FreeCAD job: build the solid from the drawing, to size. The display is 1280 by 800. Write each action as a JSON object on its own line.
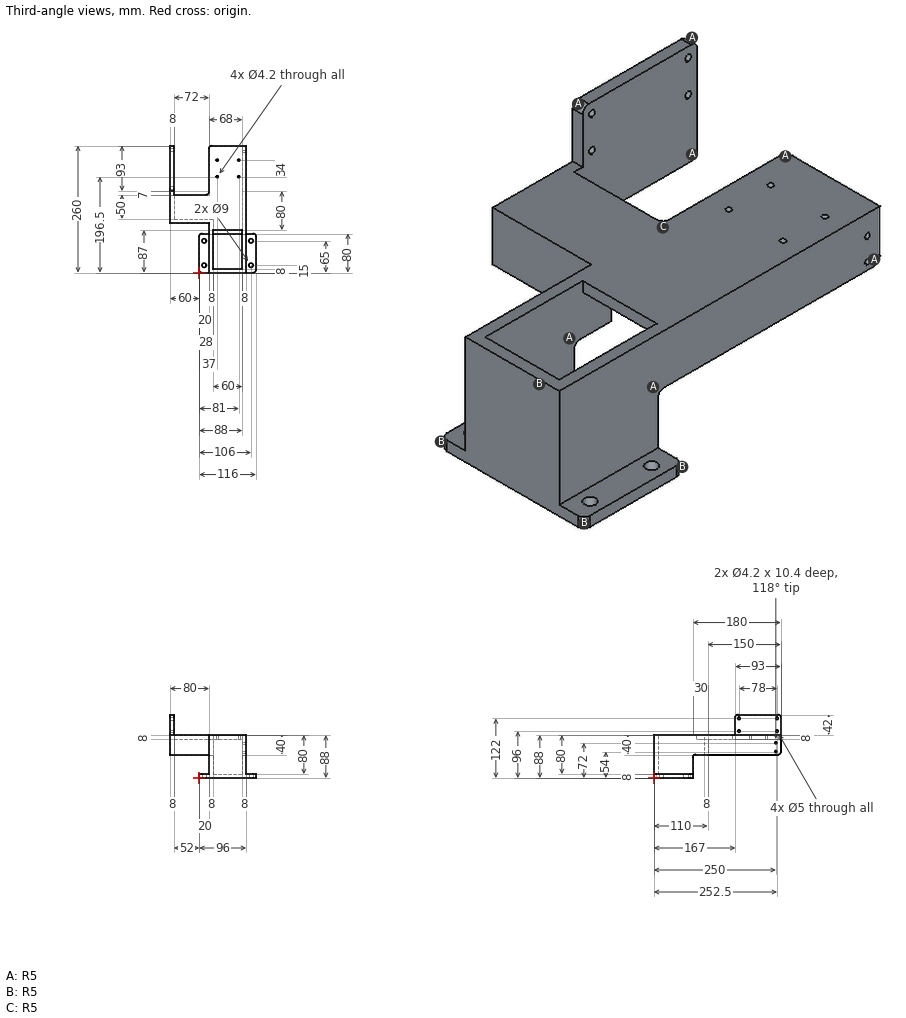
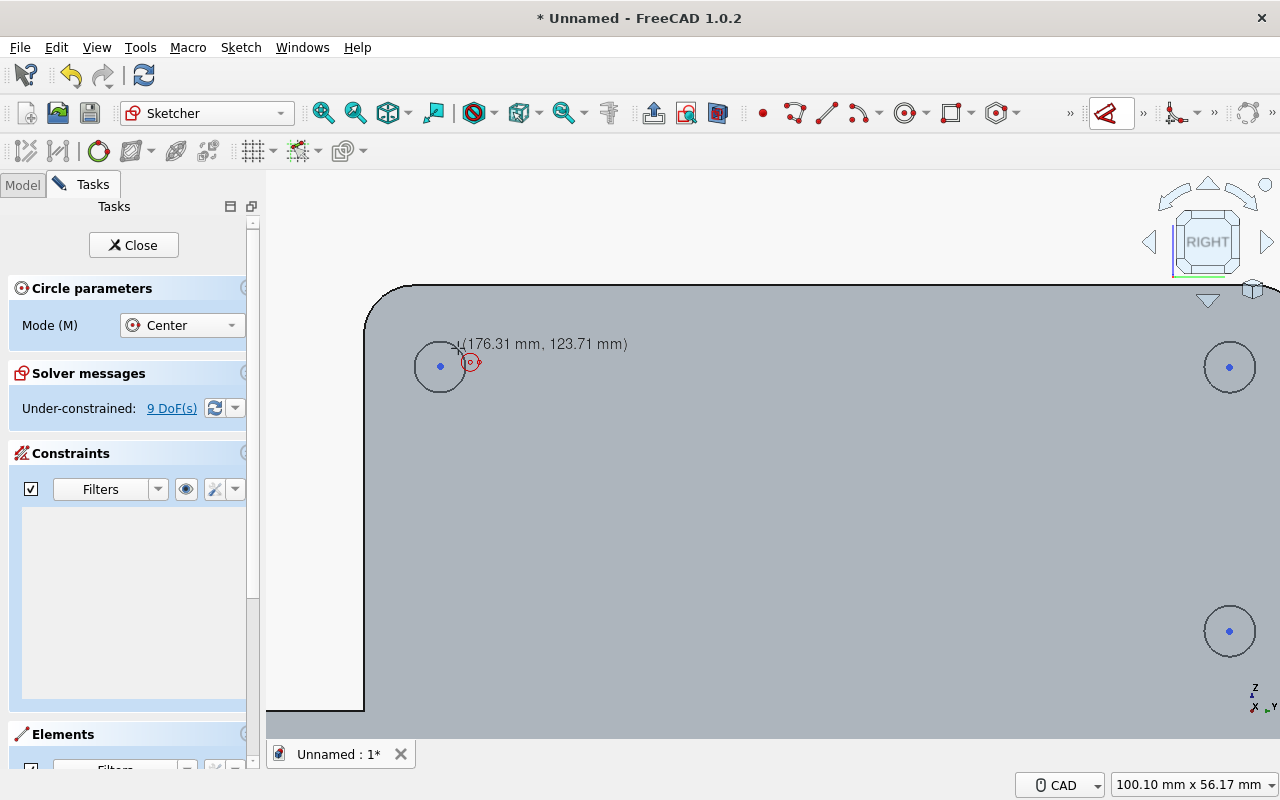
{"action": "left_click", "coordinate": [440, 630]}
{"action": "left_click", "coordinate": [458, 612]}
{"action": "key", "text": "Escape"}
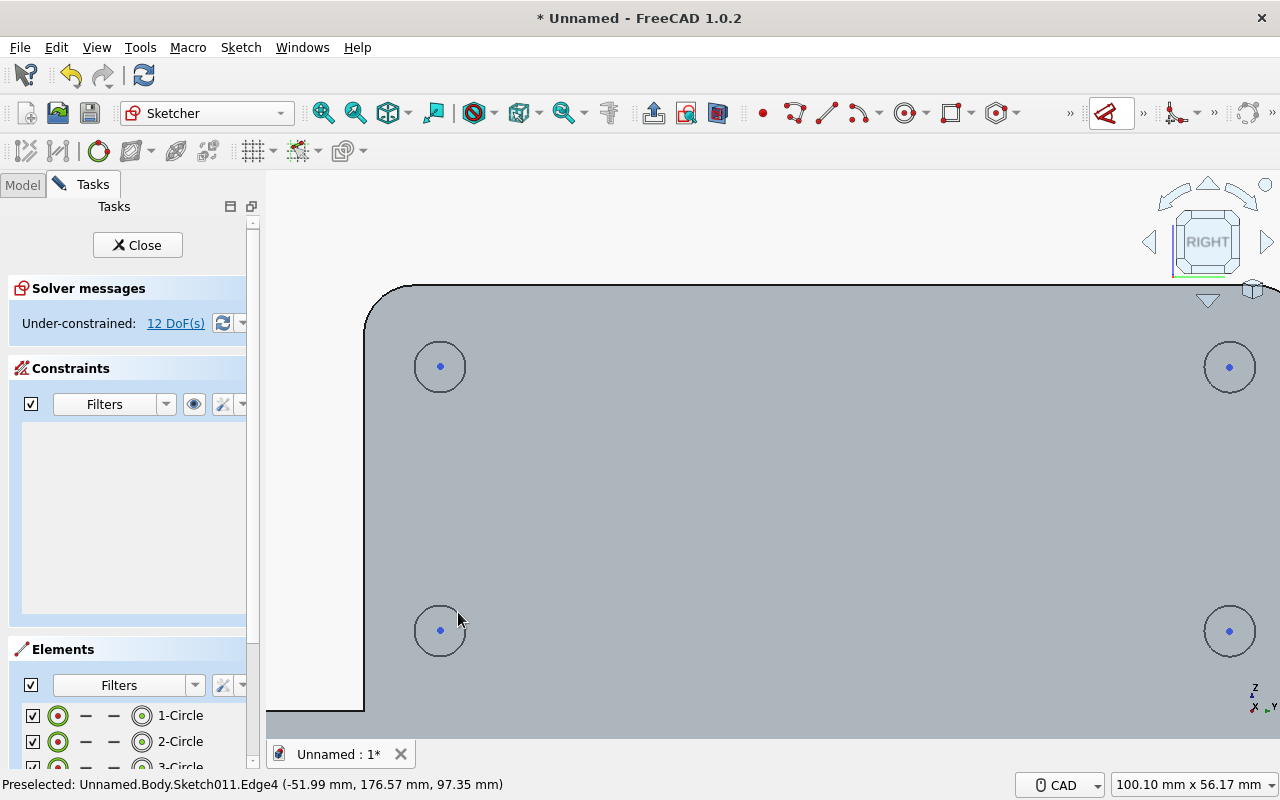
{"action": "scroll", "coordinate": [440, 366], "scroll_direction": "down", "scroll_amount": 2}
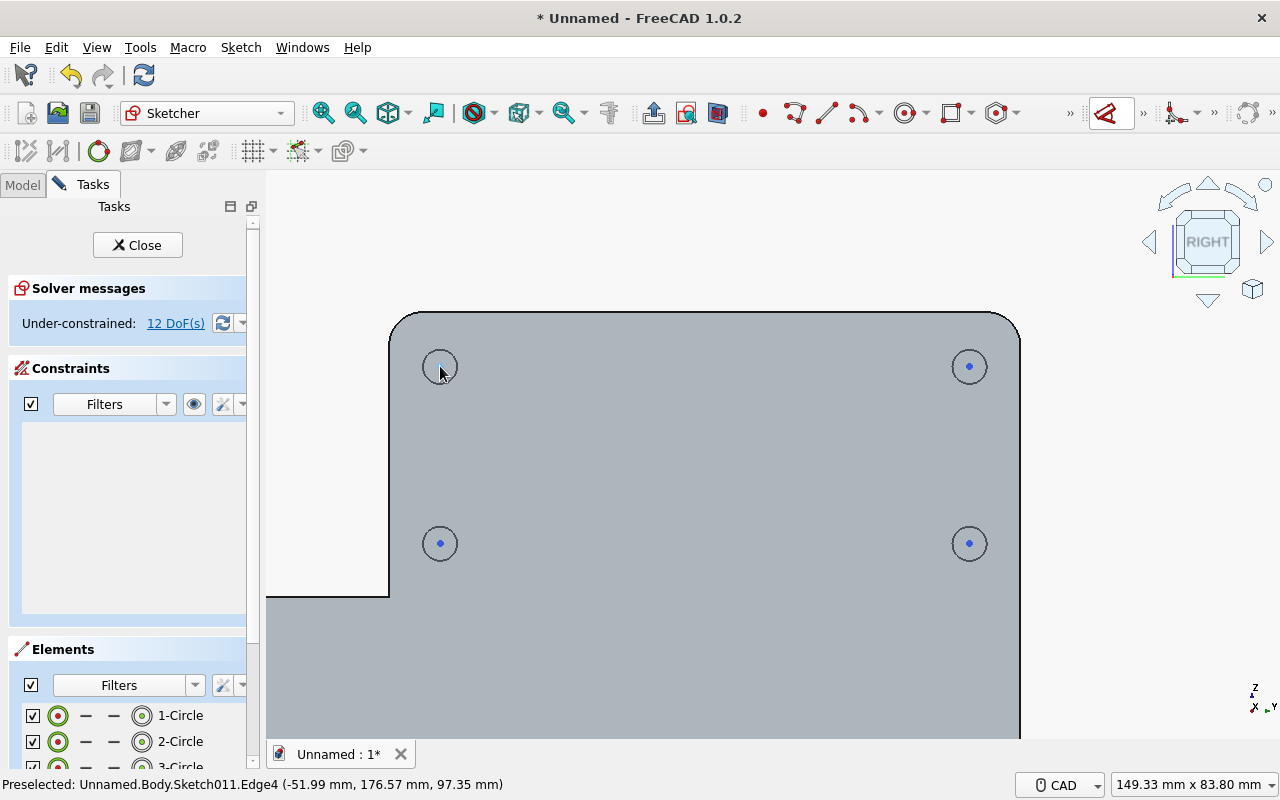
{"action": "left_click", "coordinate": [982, 532]}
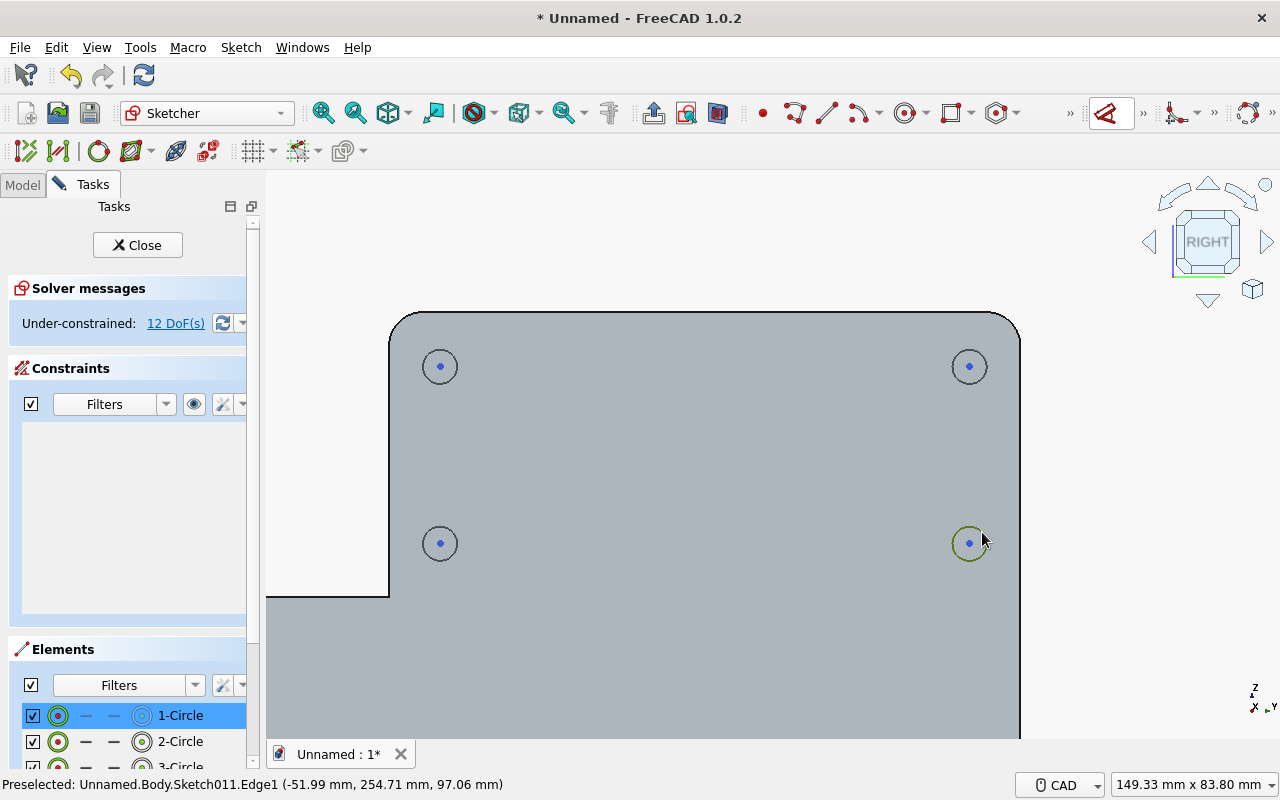
{"action": "left_click", "coordinate": [982, 355]}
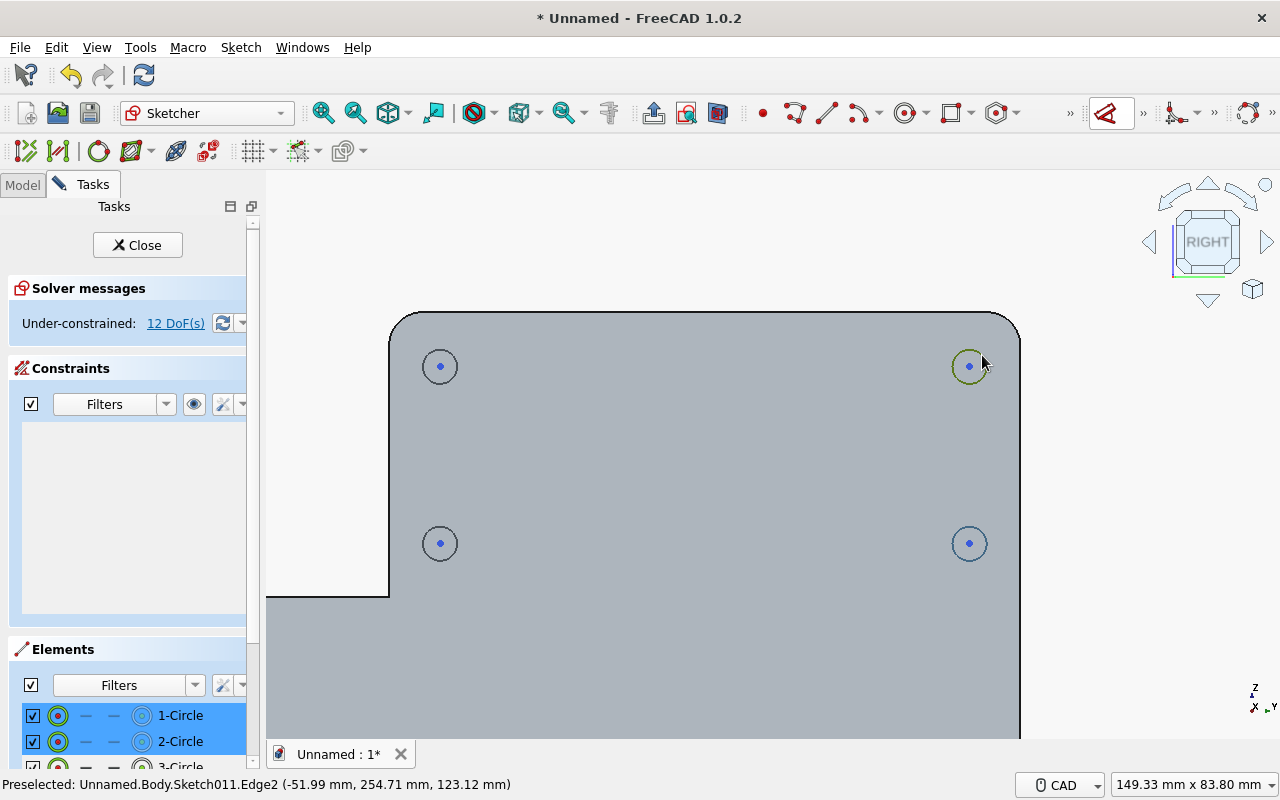
{"action": "left_click", "coordinate": [452, 355]}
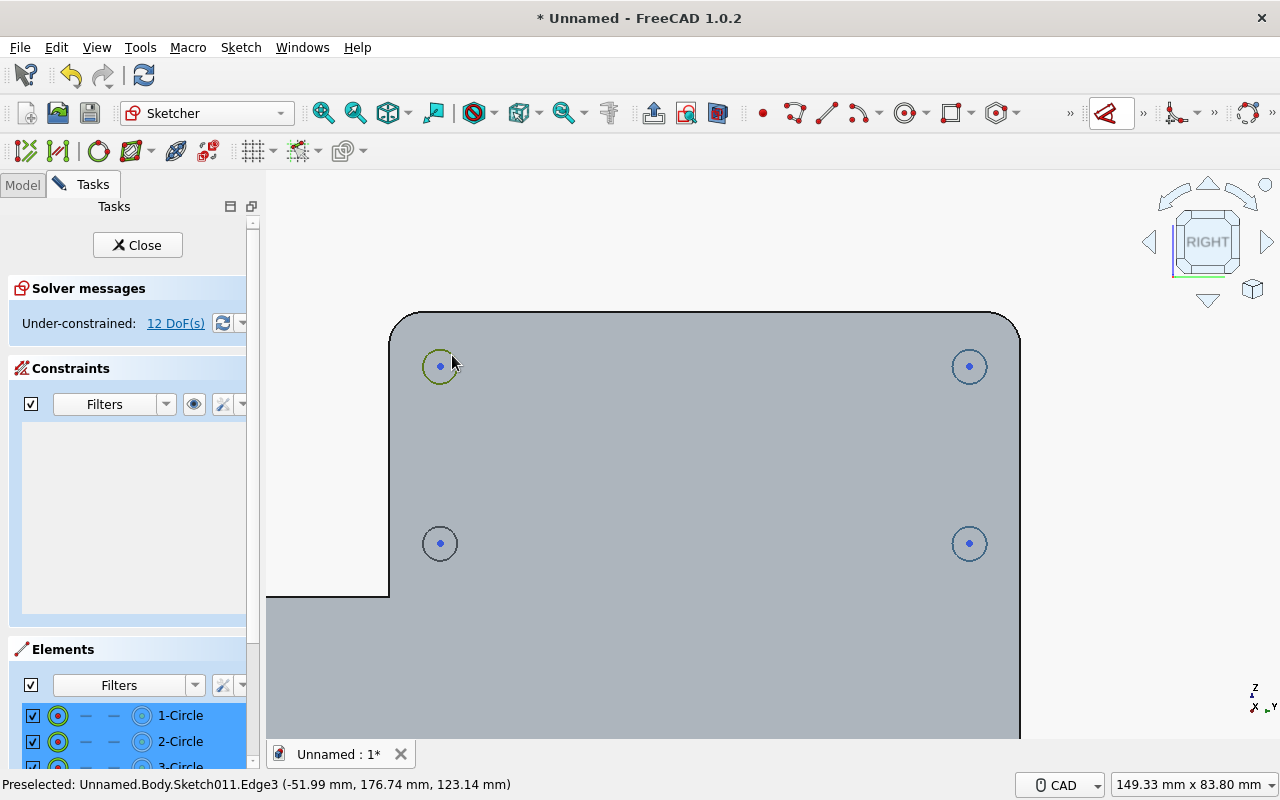
{"action": "left_click", "coordinate": [452, 532]}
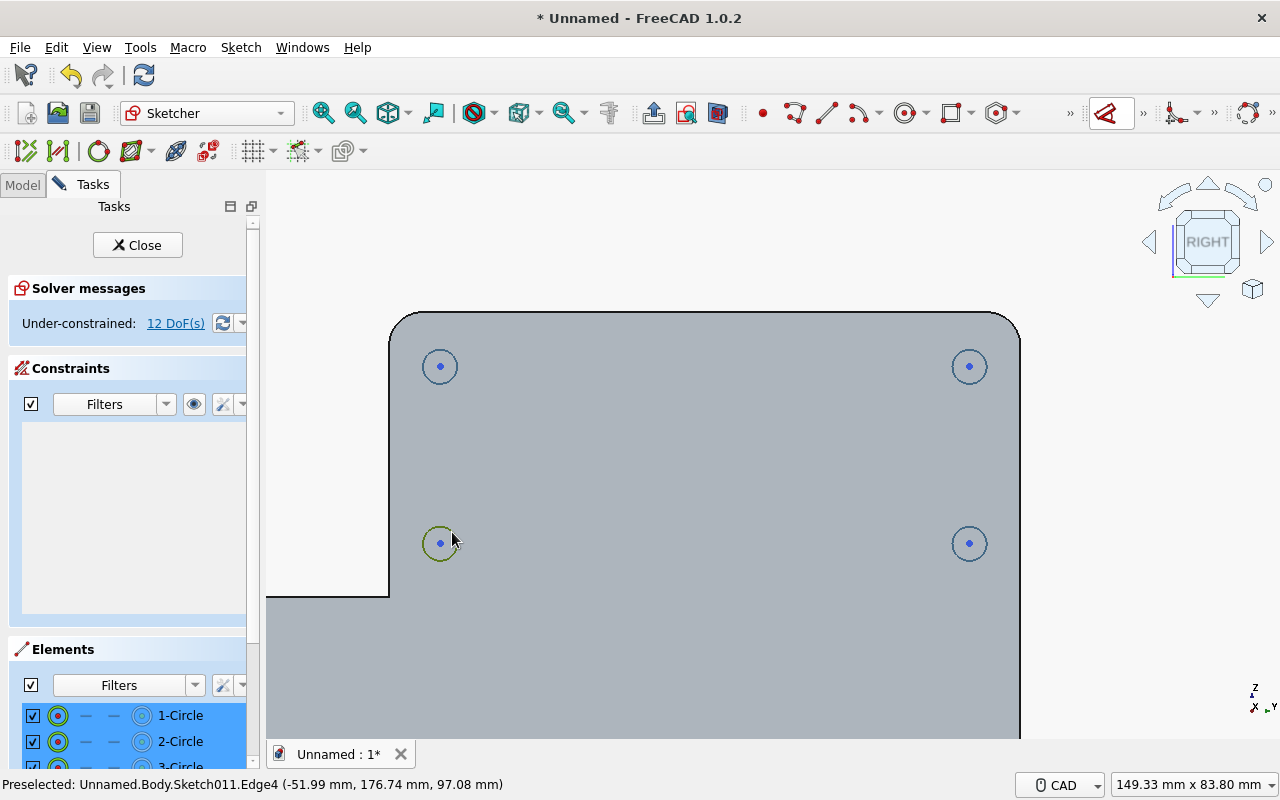
{"action": "key", "text": "e"}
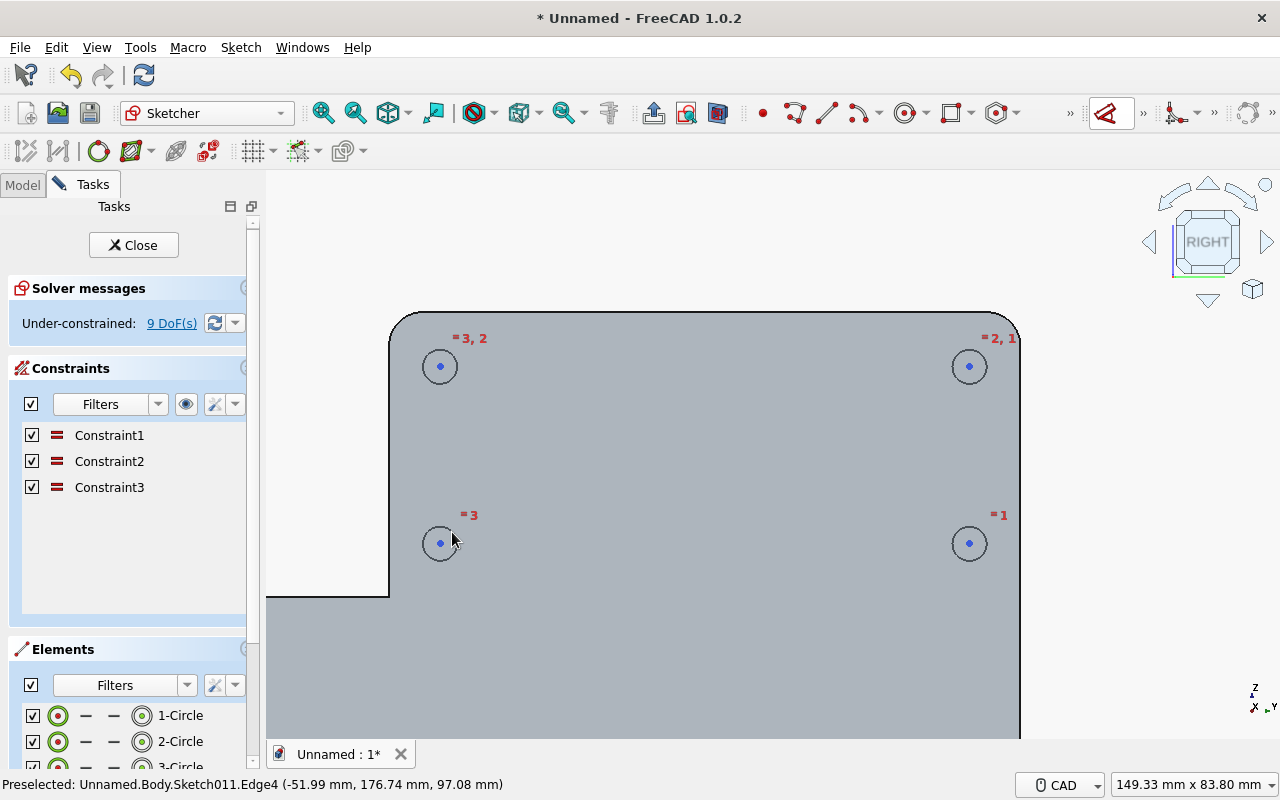
{"action": "left_click", "coordinate": [970, 544]}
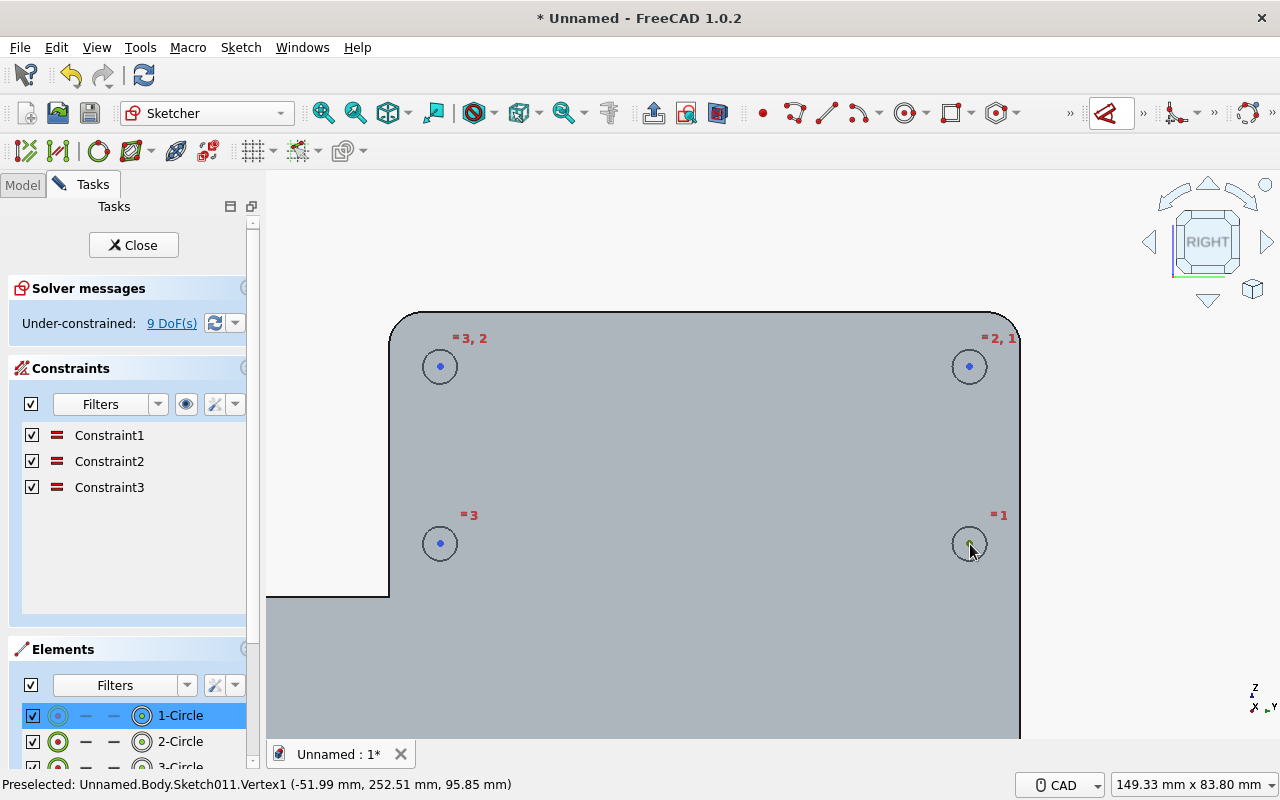
{"action": "left_click", "coordinate": [970, 367]}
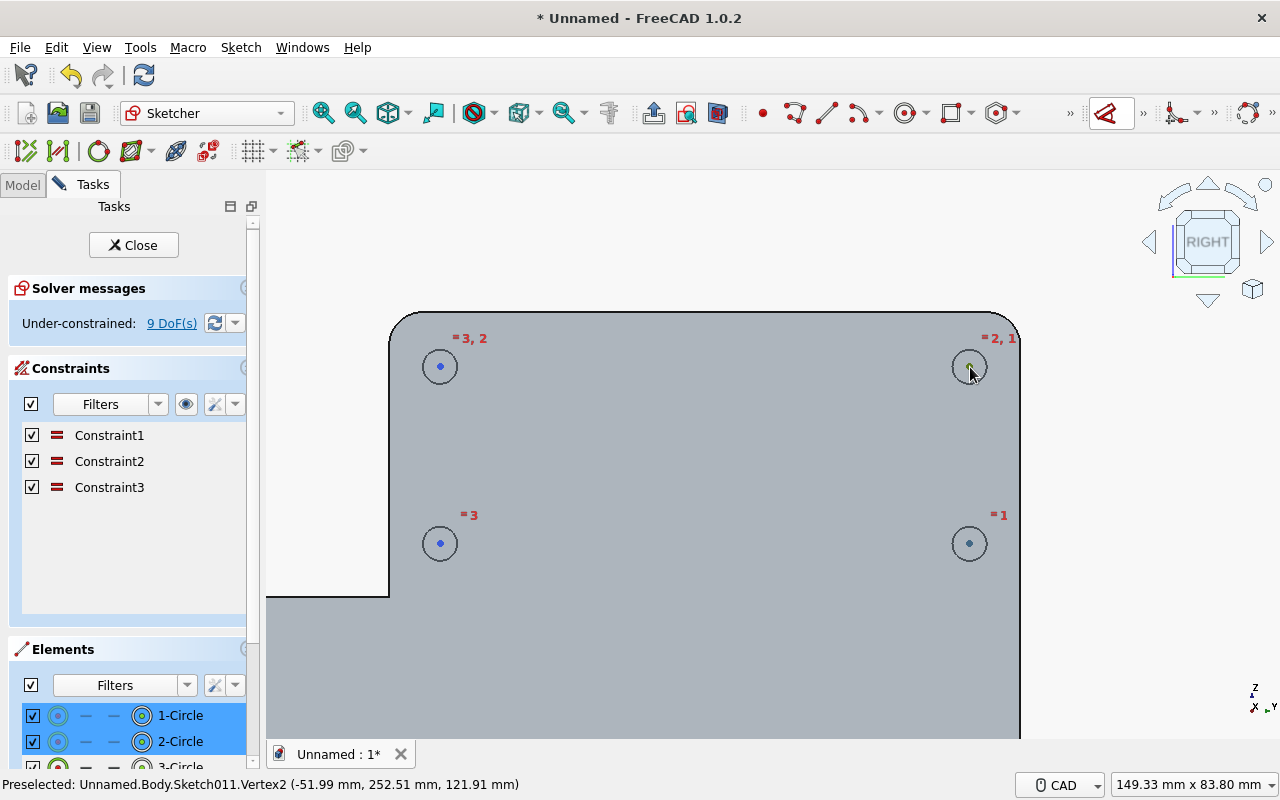
{"action": "key", "text": "v"}